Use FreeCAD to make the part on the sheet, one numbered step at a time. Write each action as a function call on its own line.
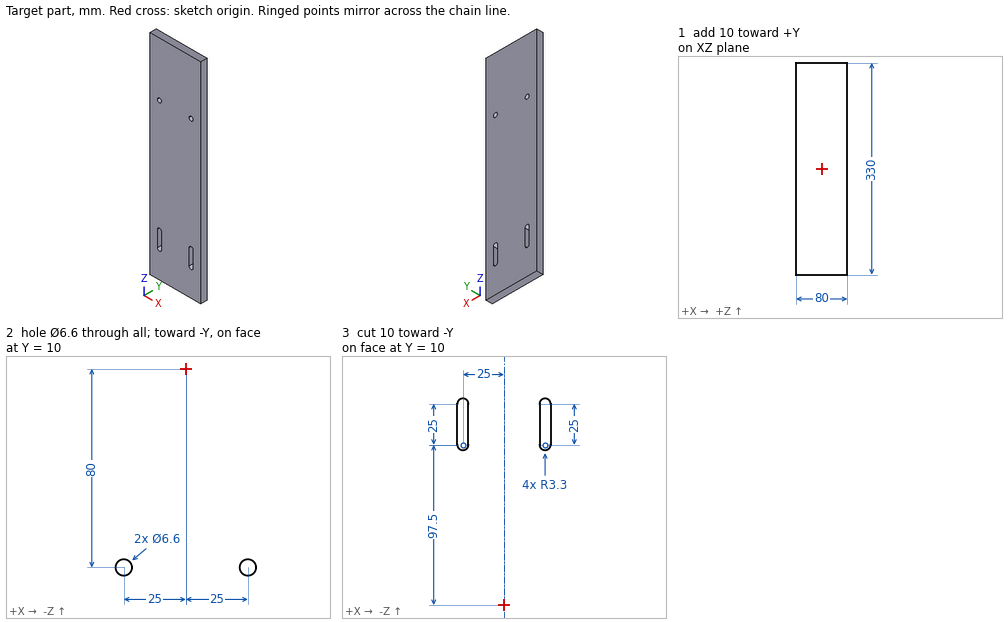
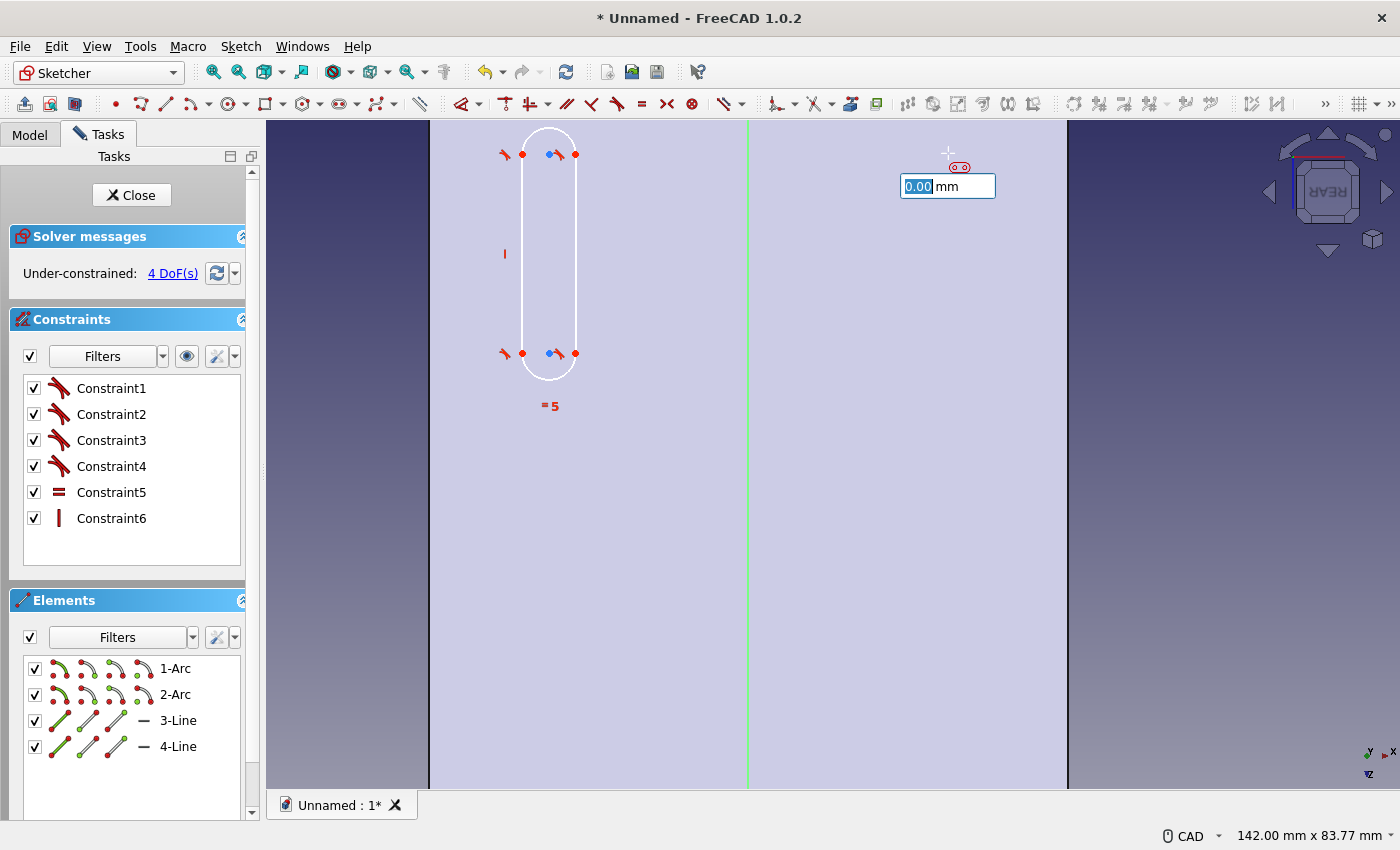
click(922, 253)
key(Escape)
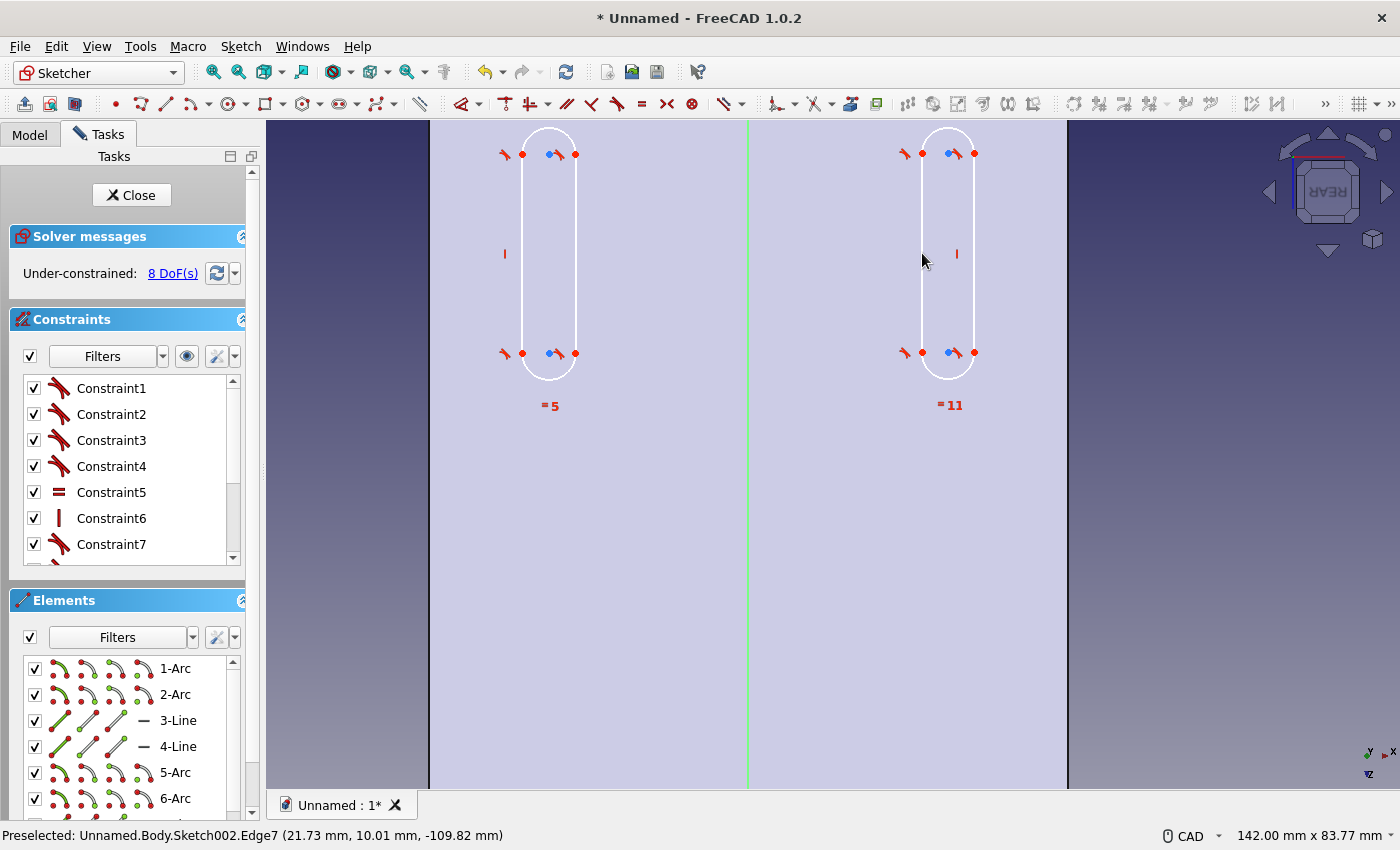
click(533, 375)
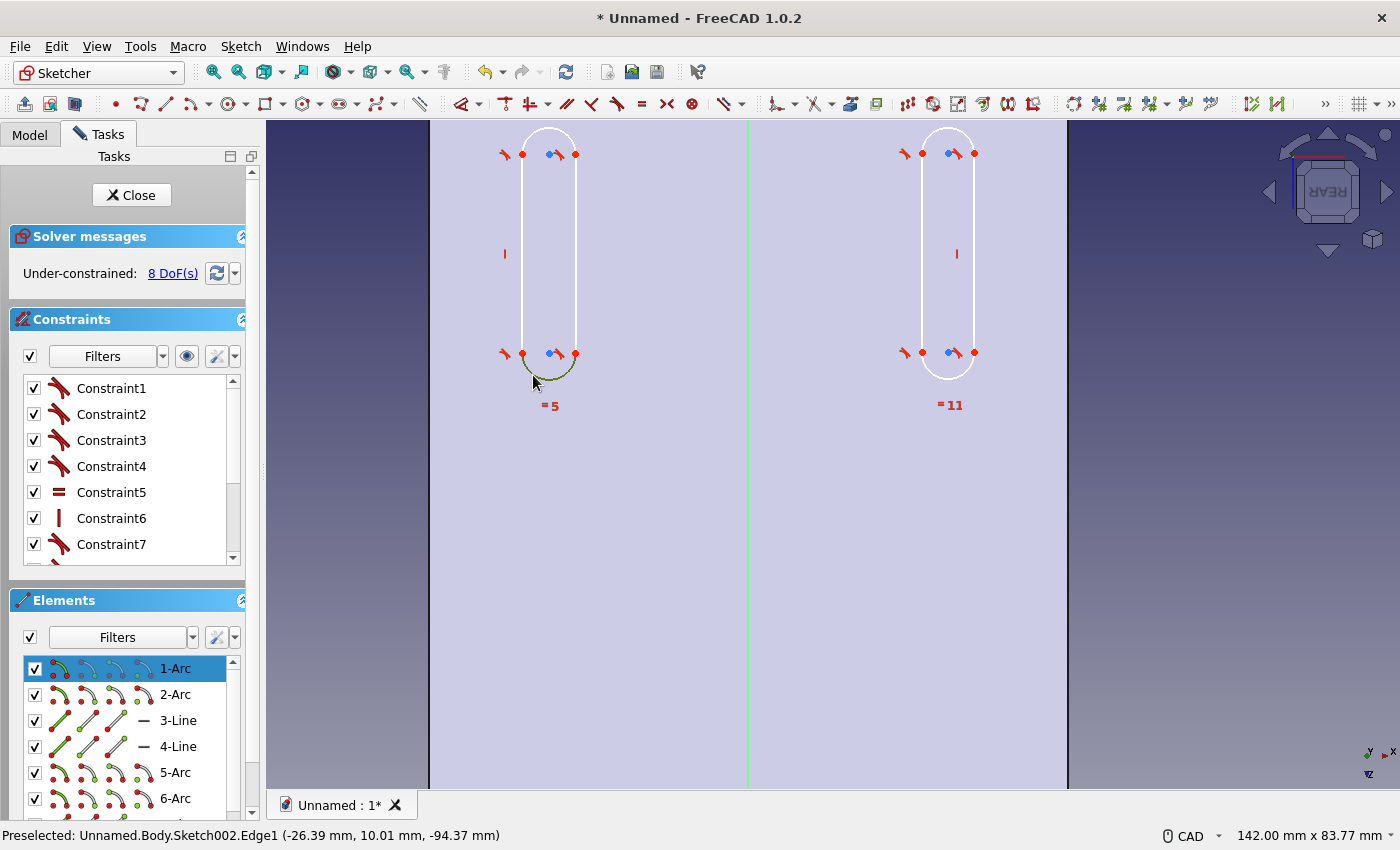
click(933, 374)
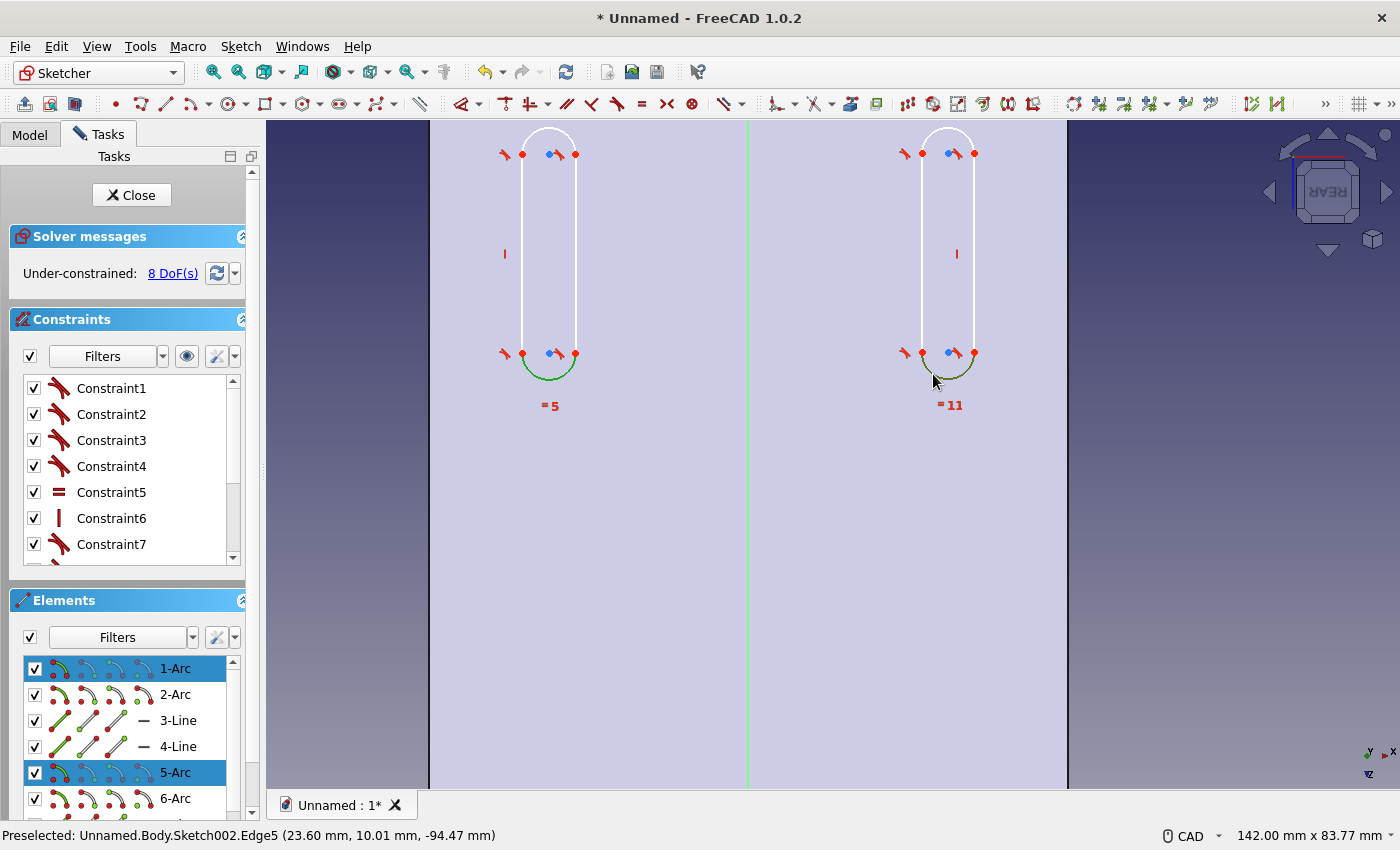
click(642, 104)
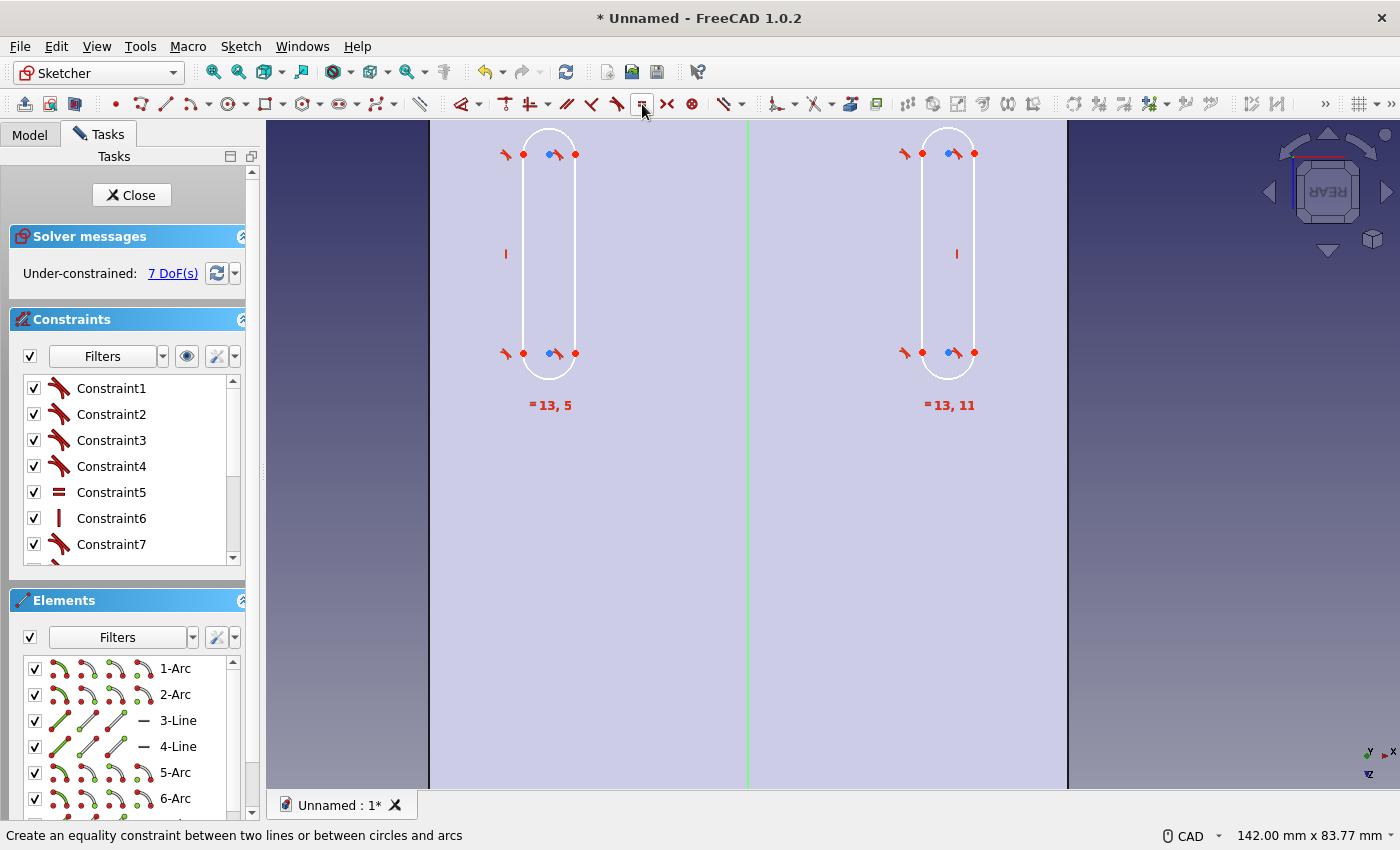
click(549, 353)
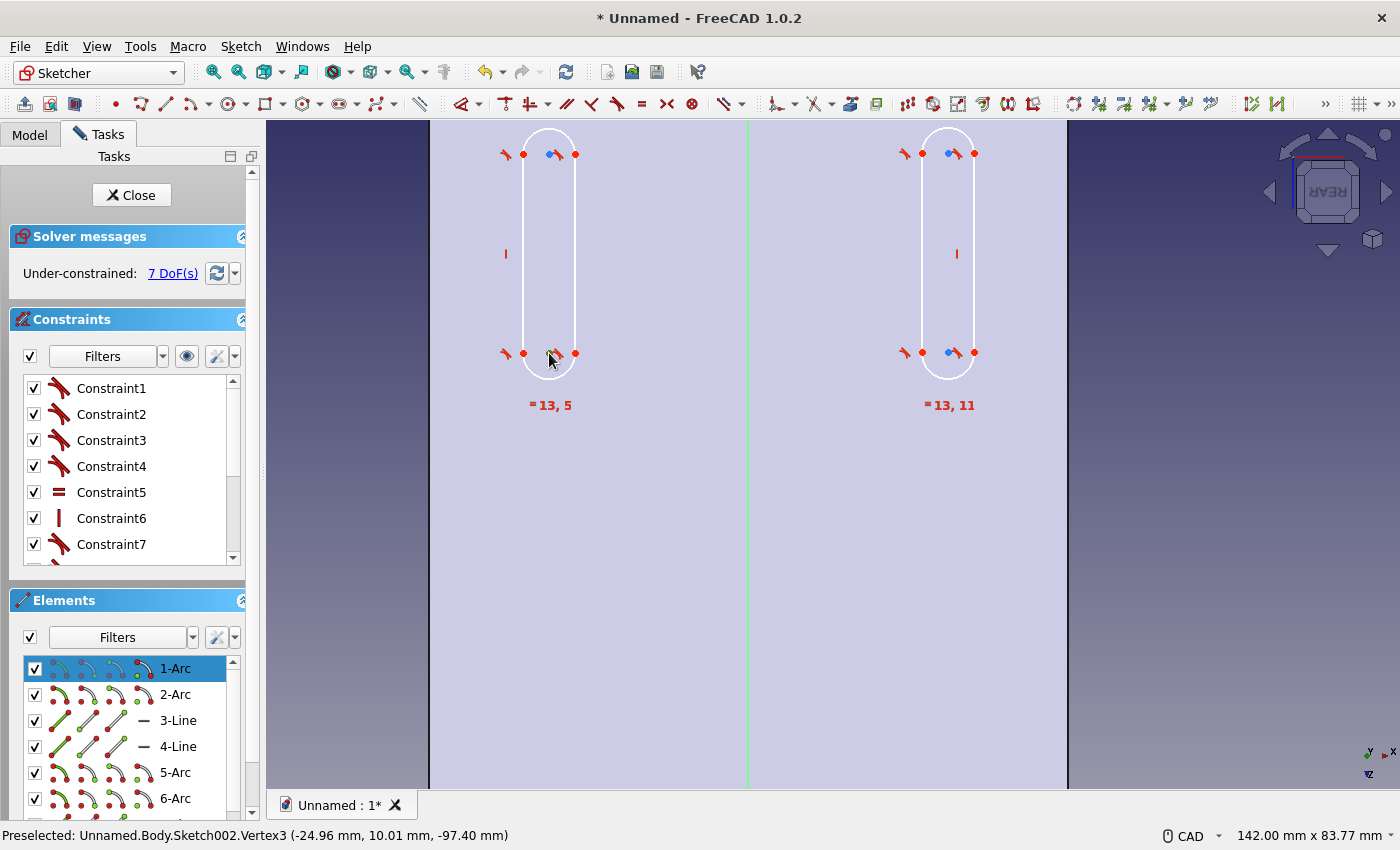
click(948, 353)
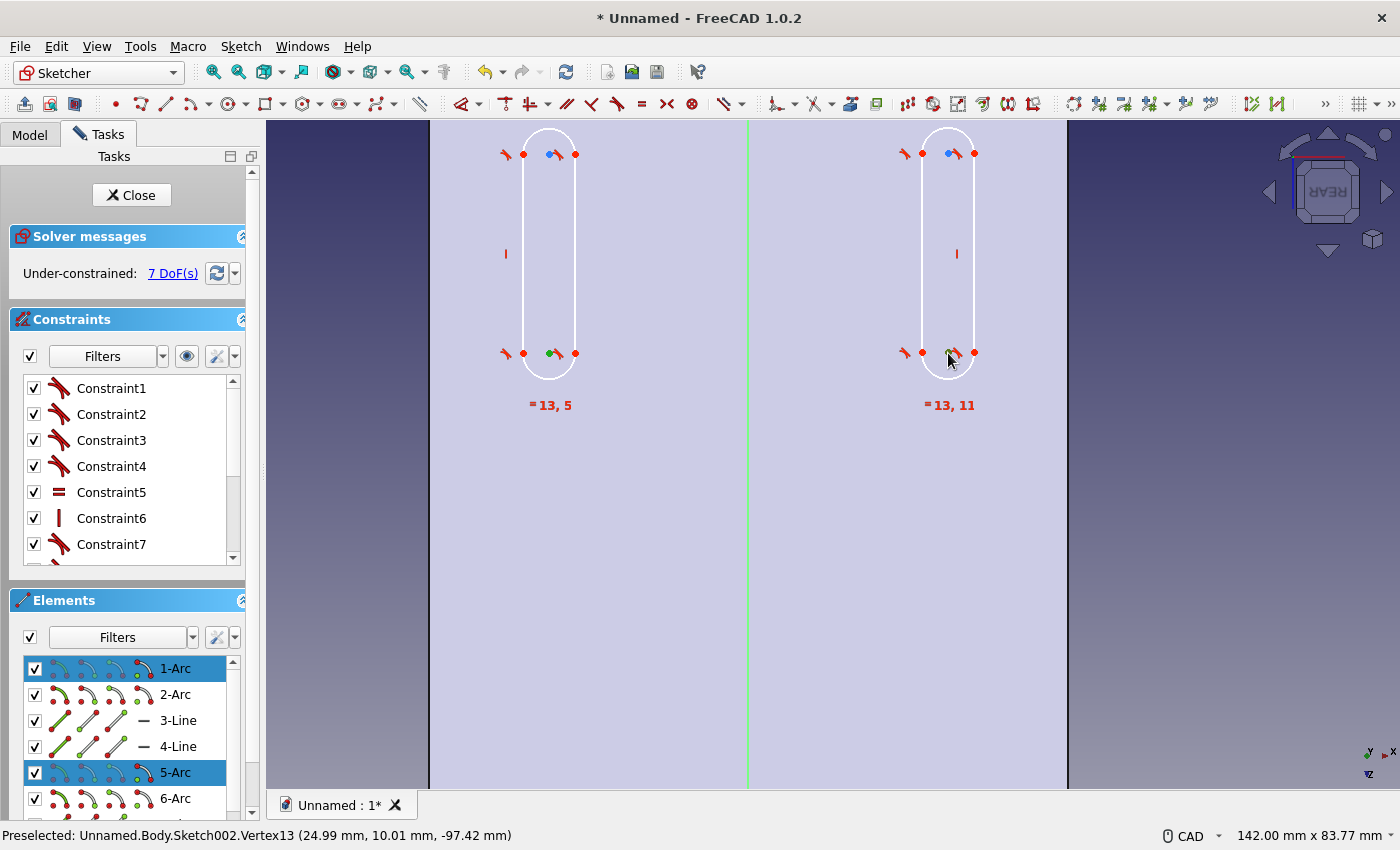
click(748, 717)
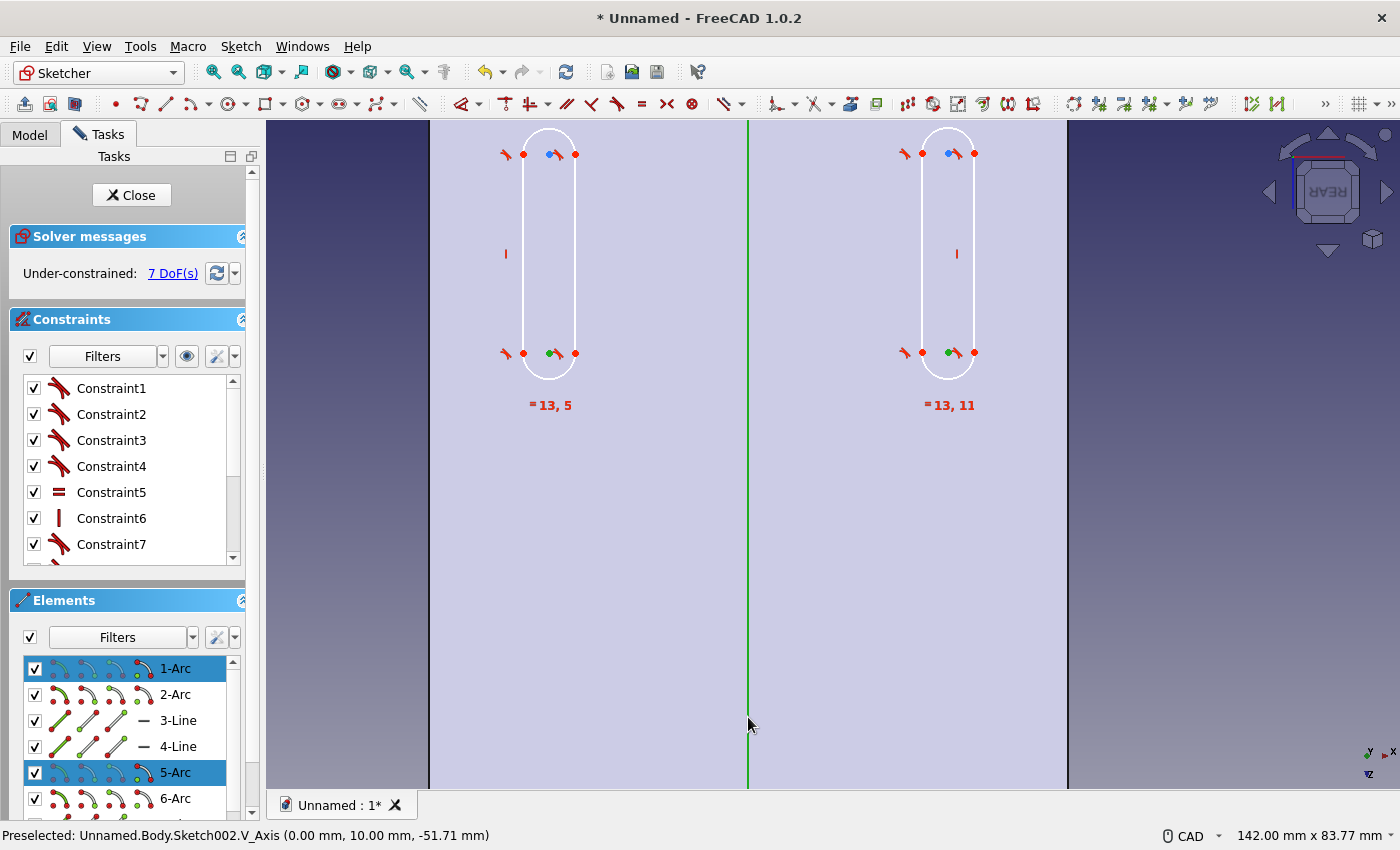
key(s)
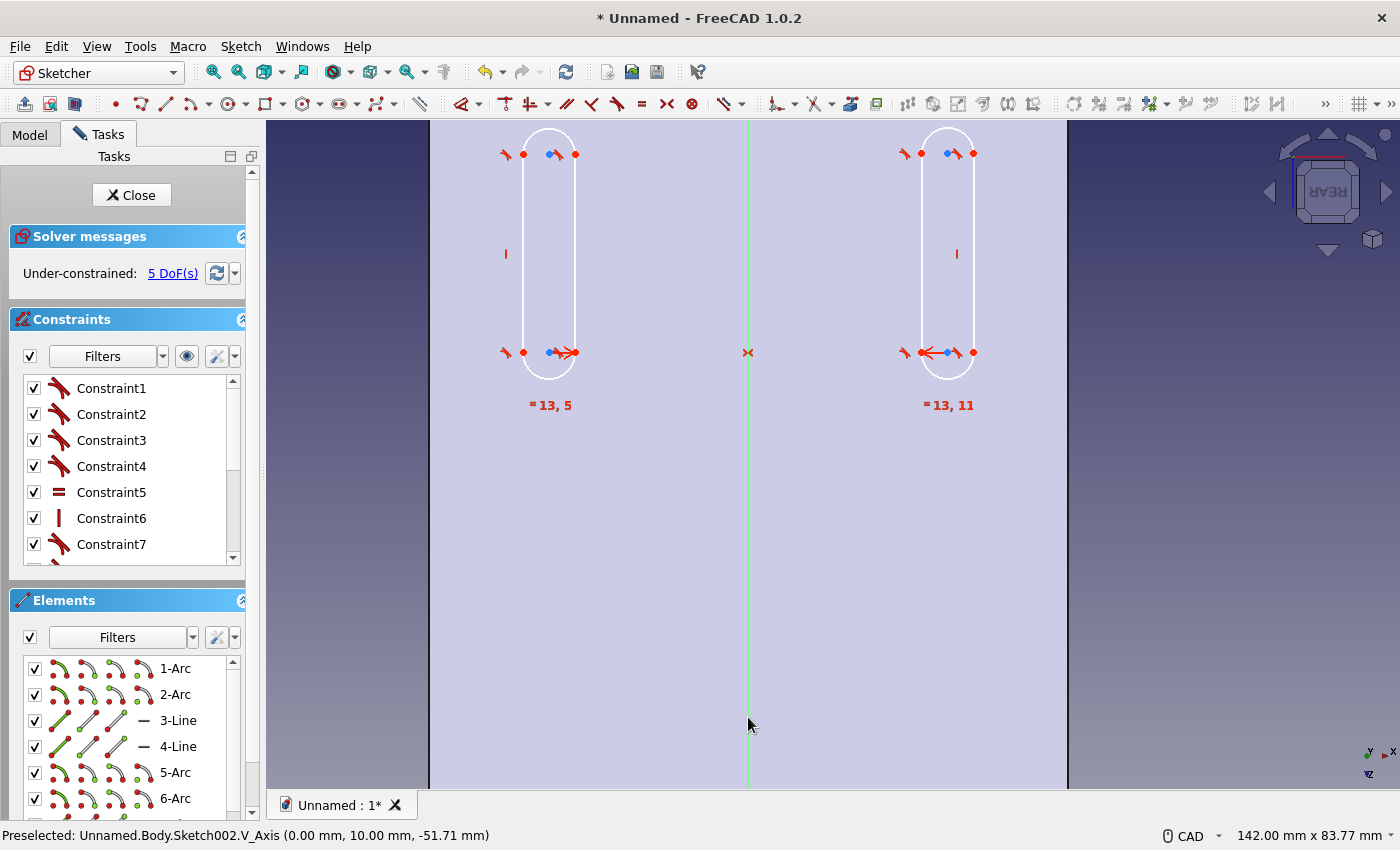
key(d)